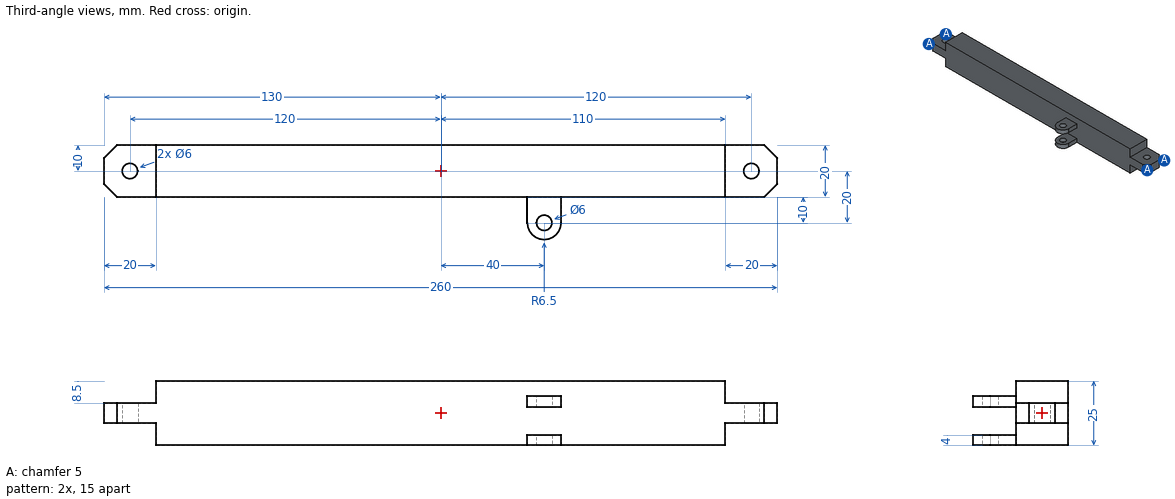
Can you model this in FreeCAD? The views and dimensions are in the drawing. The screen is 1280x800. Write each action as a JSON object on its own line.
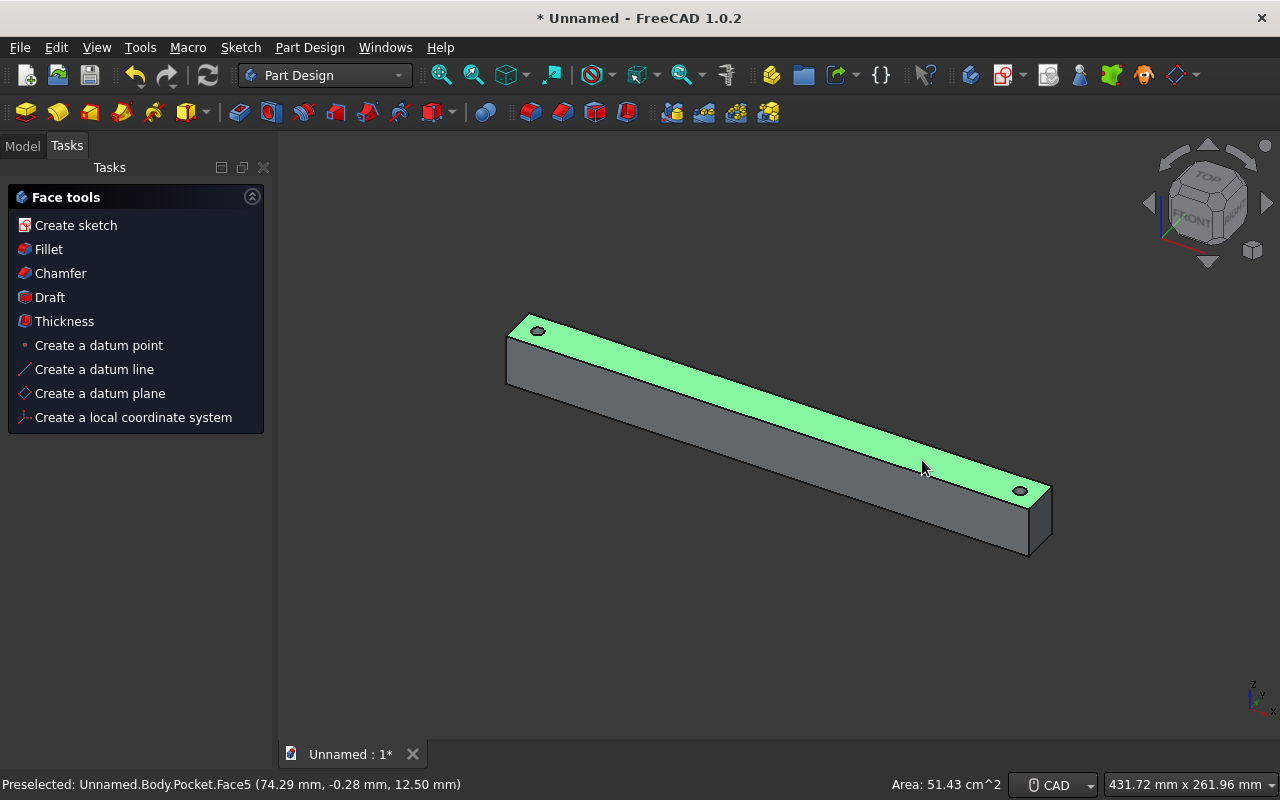
{"action": "left_click", "coordinate": [1004, 76]}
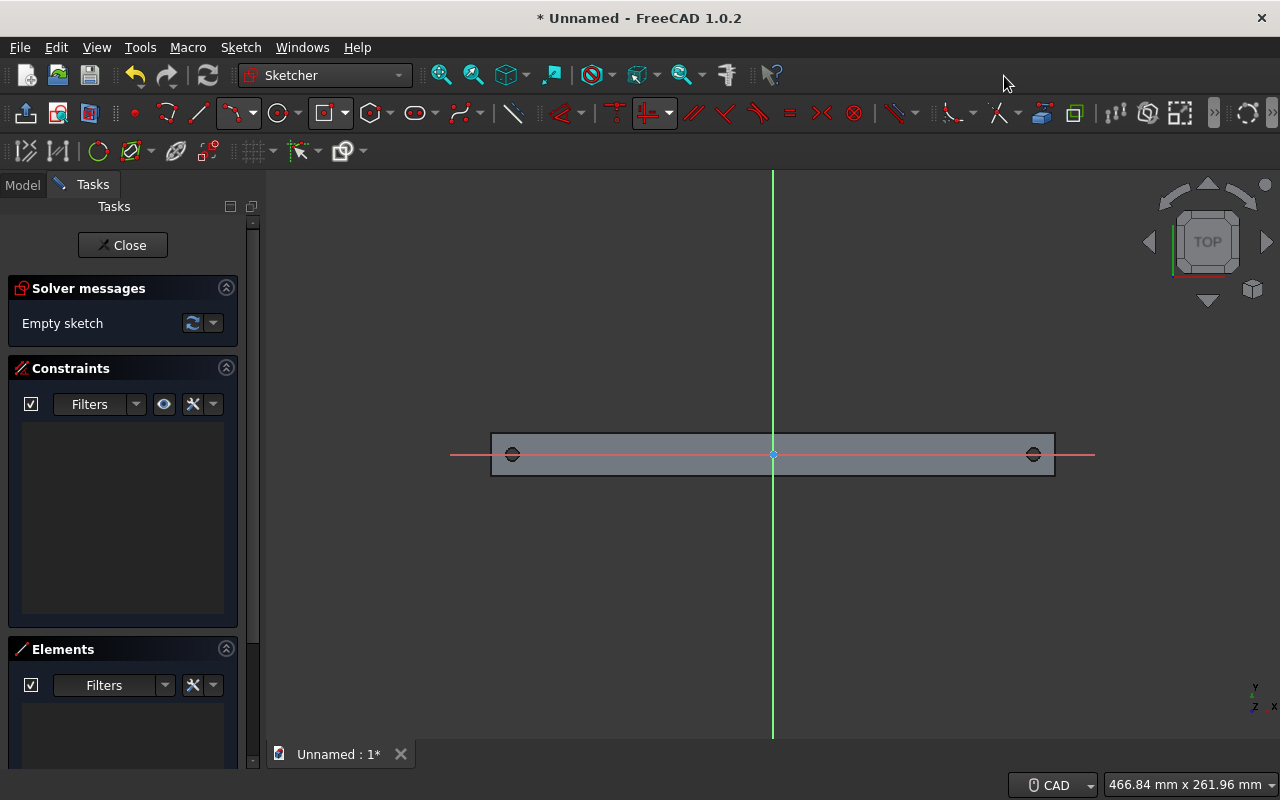
{"action": "key", "text": "g r"}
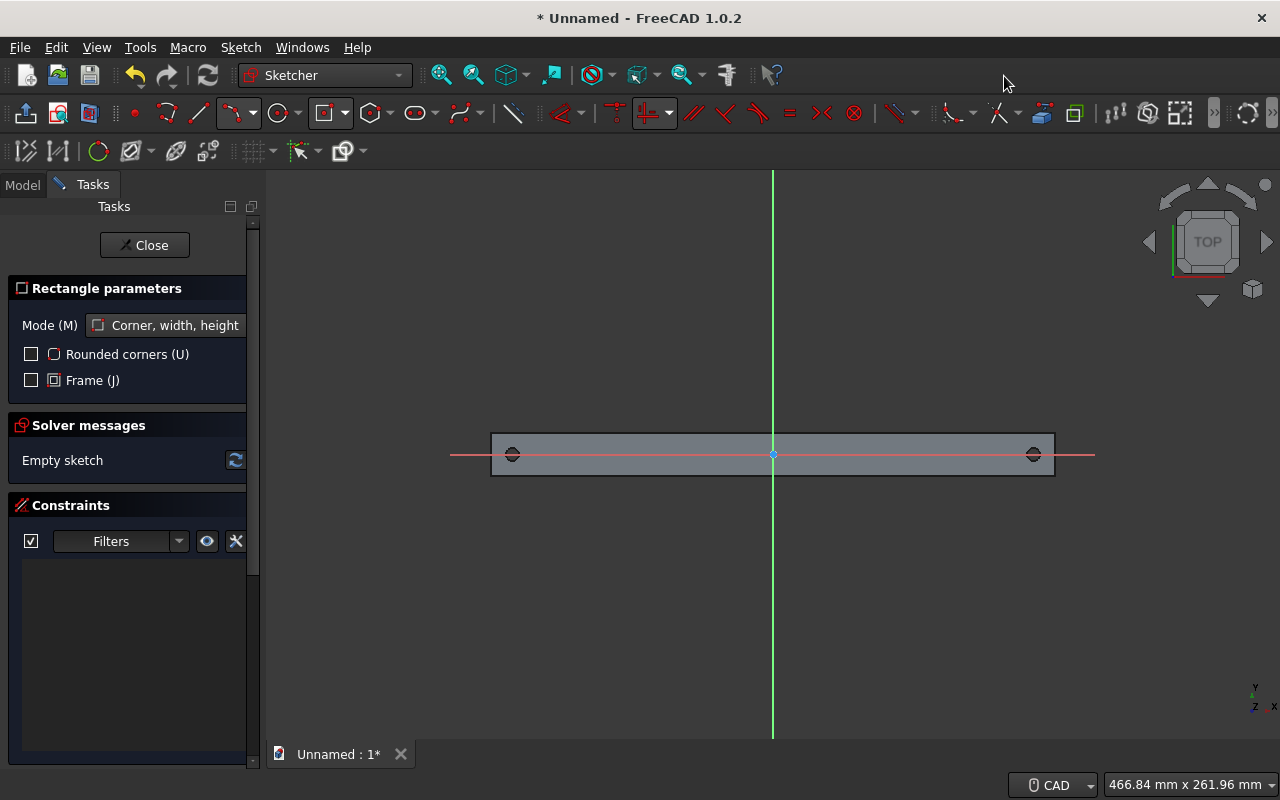
{"action": "left_click", "coordinate": [491, 433]}
{"action": "mouse_move", "coordinate": [534, 476]}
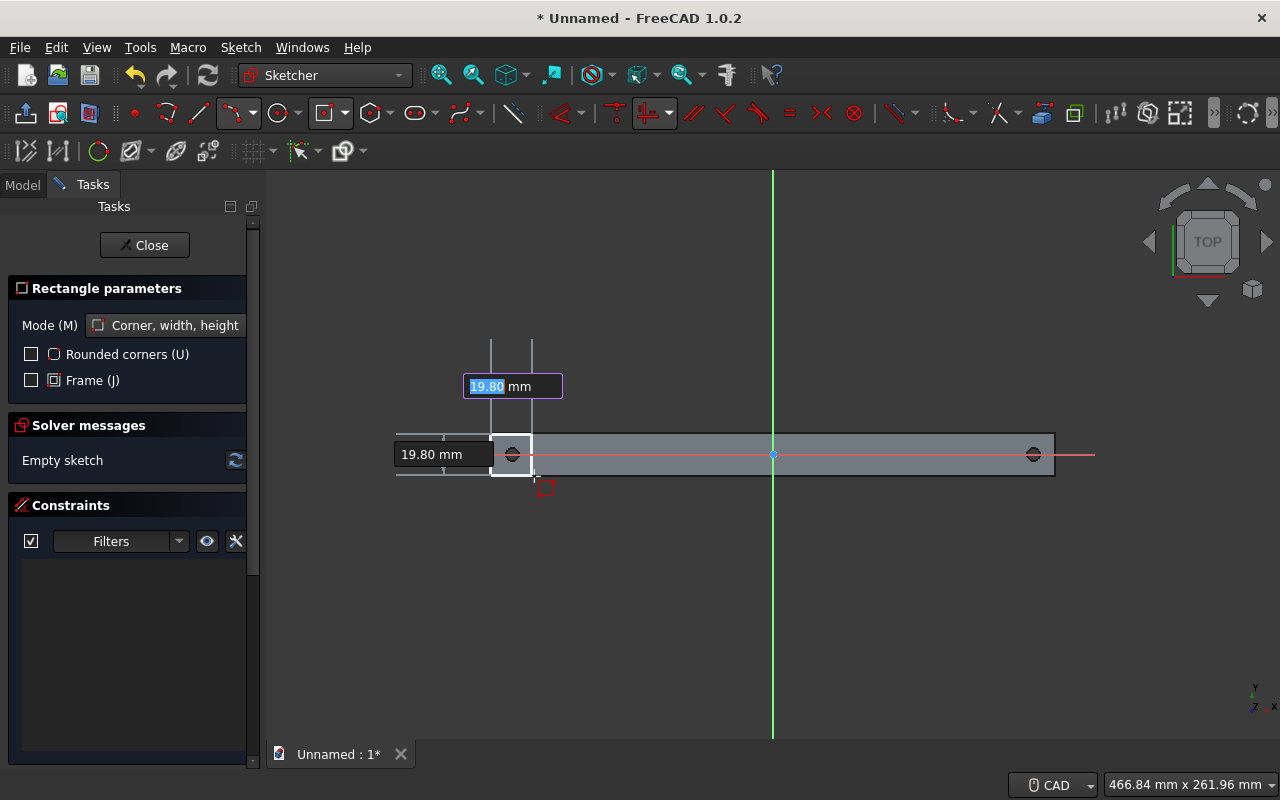
{"action": "type", "text": "20"}
{"action": "key", "text": "Tab"}
{"action": "type", "text": "20"}
{"action": "key", "text": "Return"}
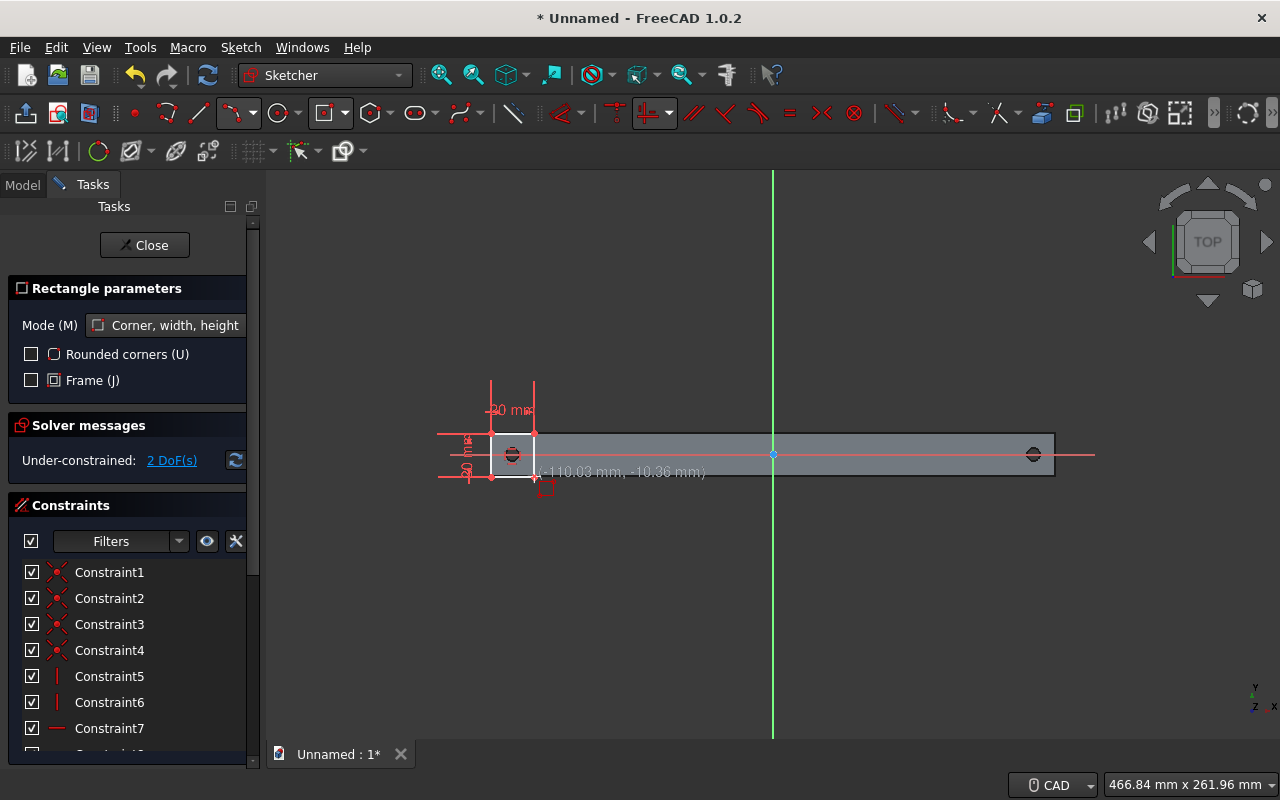
{"action": "left_click", "coordinate": [1012, 433]}
{"action": "mouse_move", "coordinate": [1055, 476]}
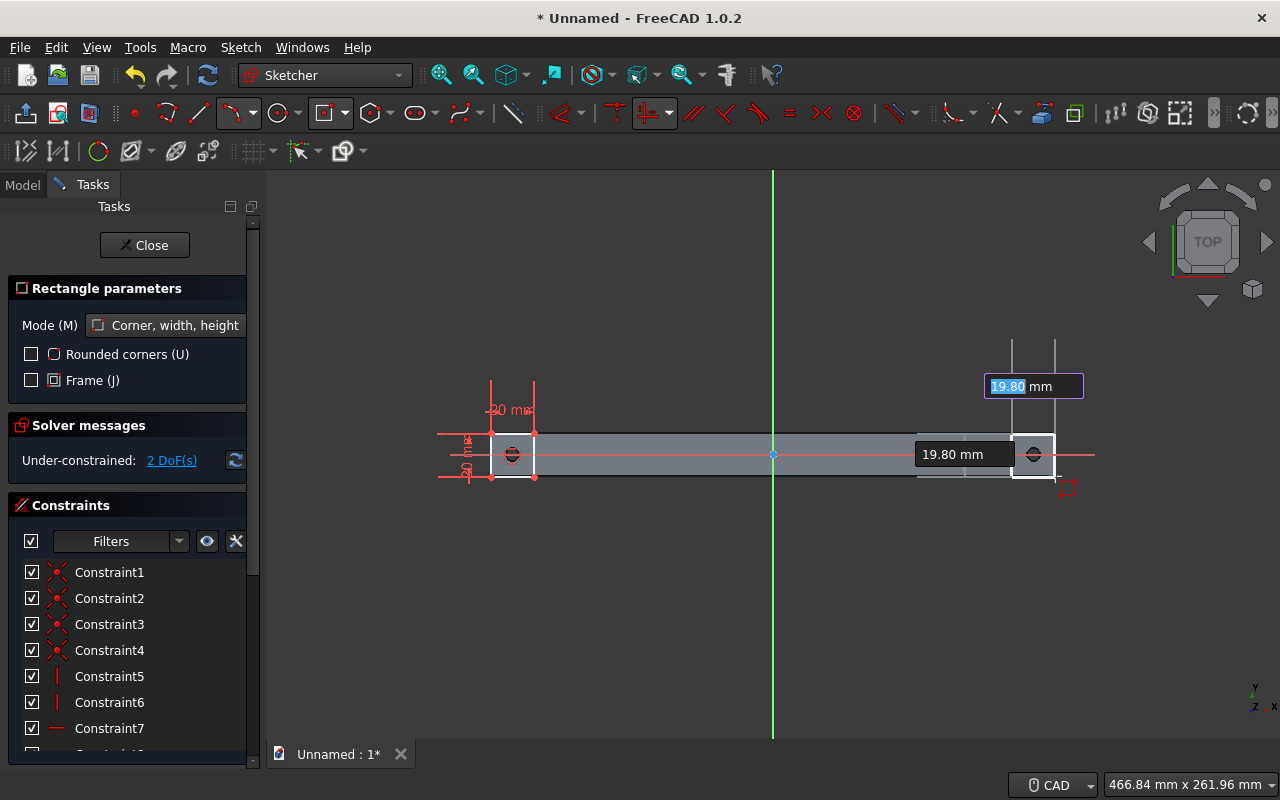
{"action": "type", "text": "20"}
{"action": "key", "text": "Tab"}
{"action": "type", "text": "20"}
{"action": "key", "text": "Return"}
{"action": "key", "text": "Escape"}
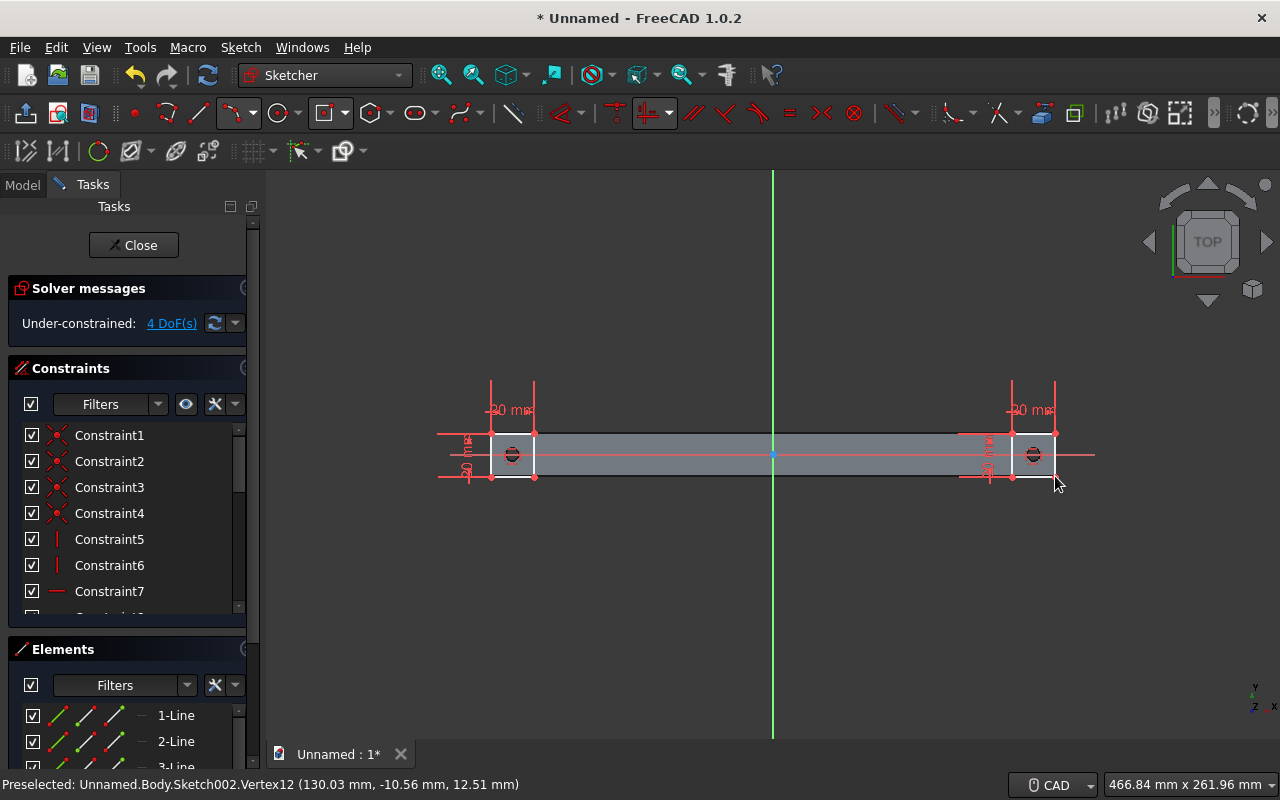
{"action": "key", "text": "d"}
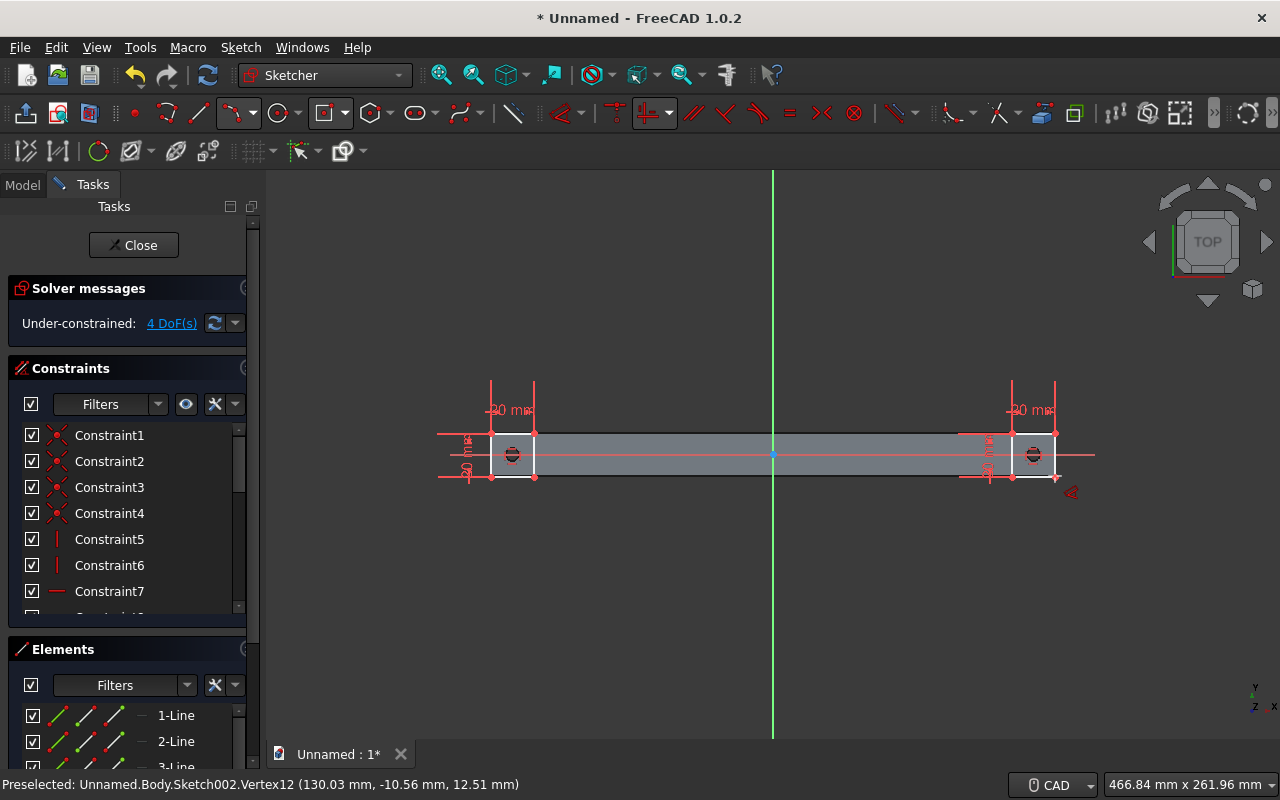
{"action": "scroll", "coordinate": [491, 434], "scroll_direction": "up", "scroll_amount": 4}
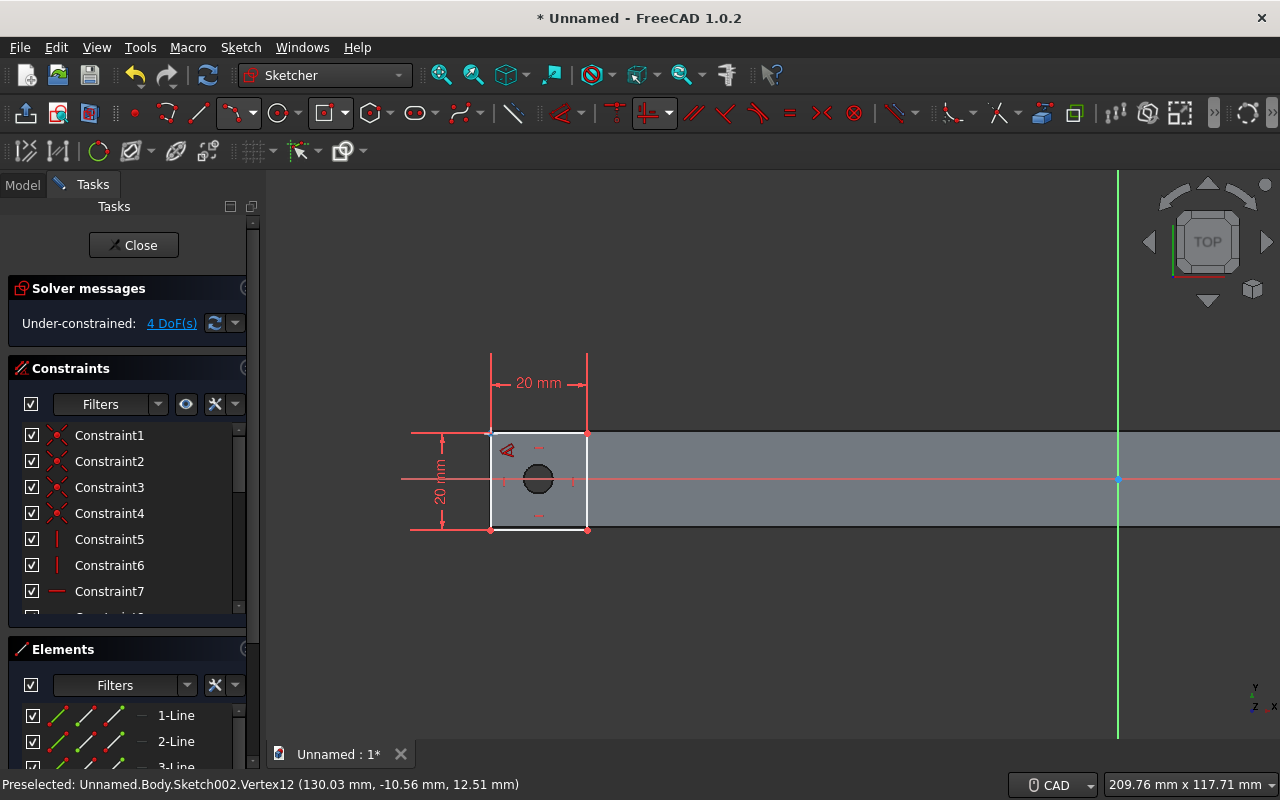
{"action": "left_click", "coordinate": [491, 433]}
{"action": "left_click", "coordinate": [457, 456]}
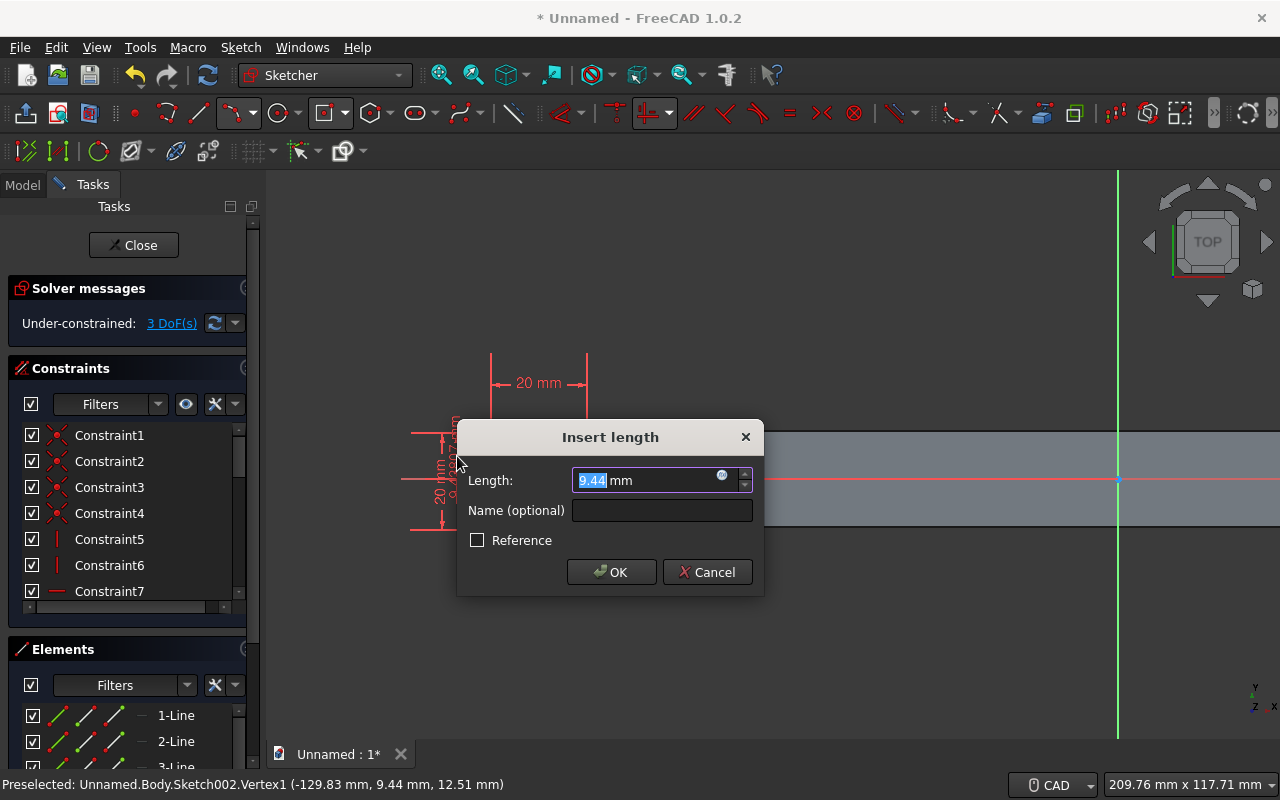
{"action": "type", "text": "10"}
{"action": "key", "text": "Return"}